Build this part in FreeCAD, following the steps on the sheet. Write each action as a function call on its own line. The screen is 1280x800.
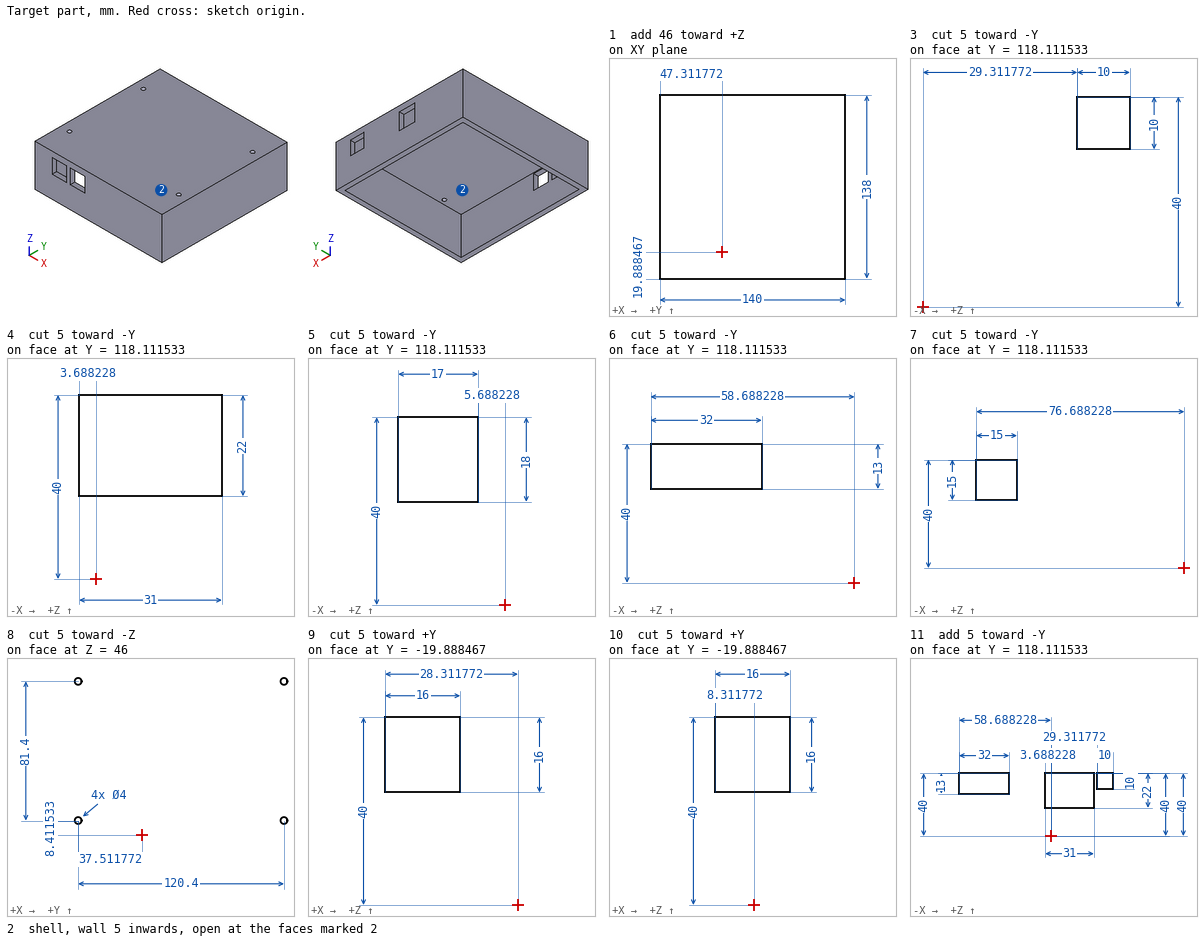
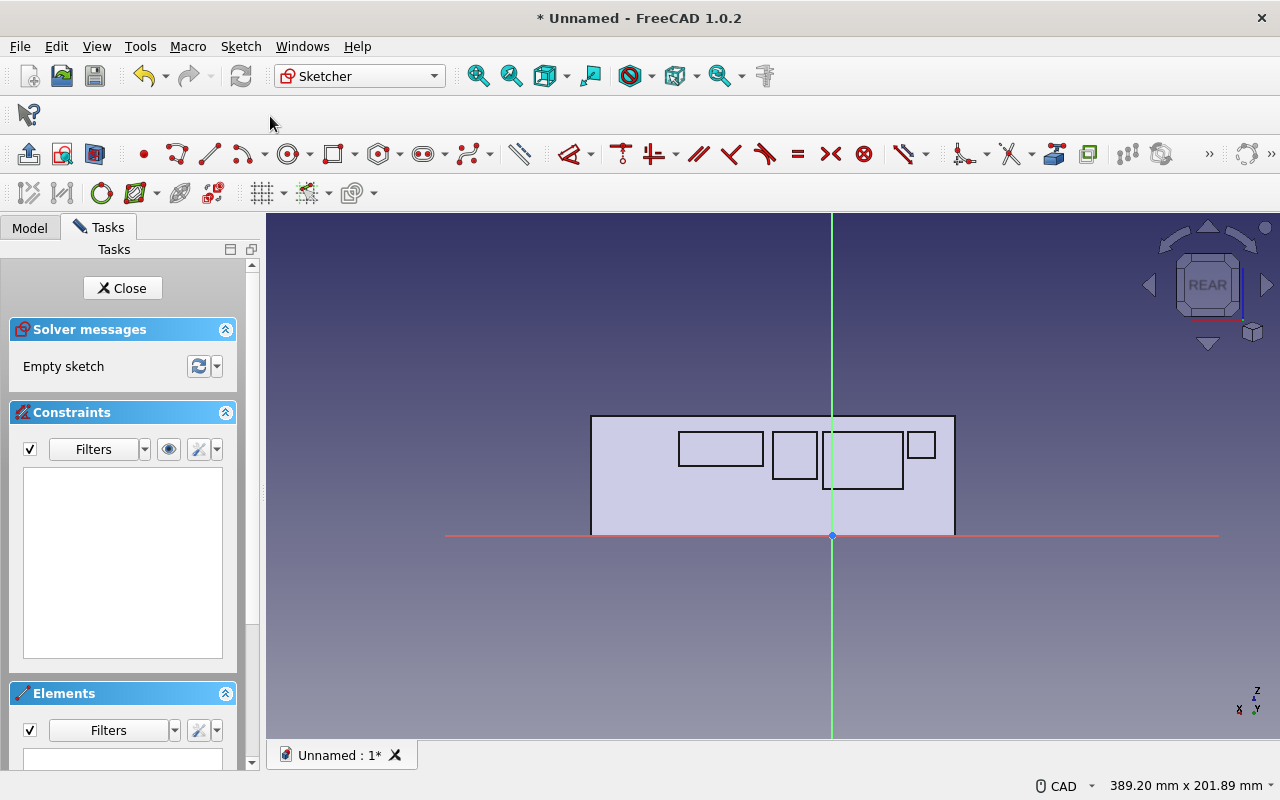
scroll(645, 448, up, 11)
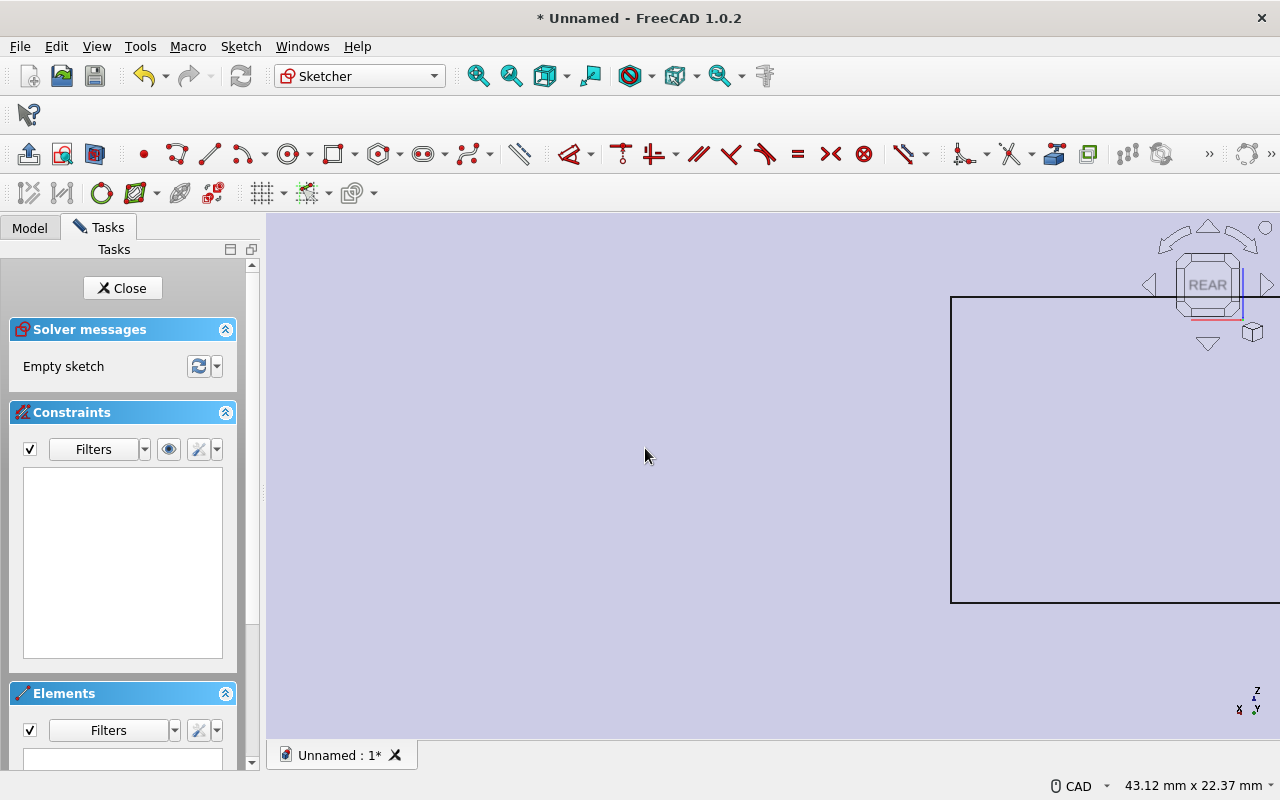
click(332, 154)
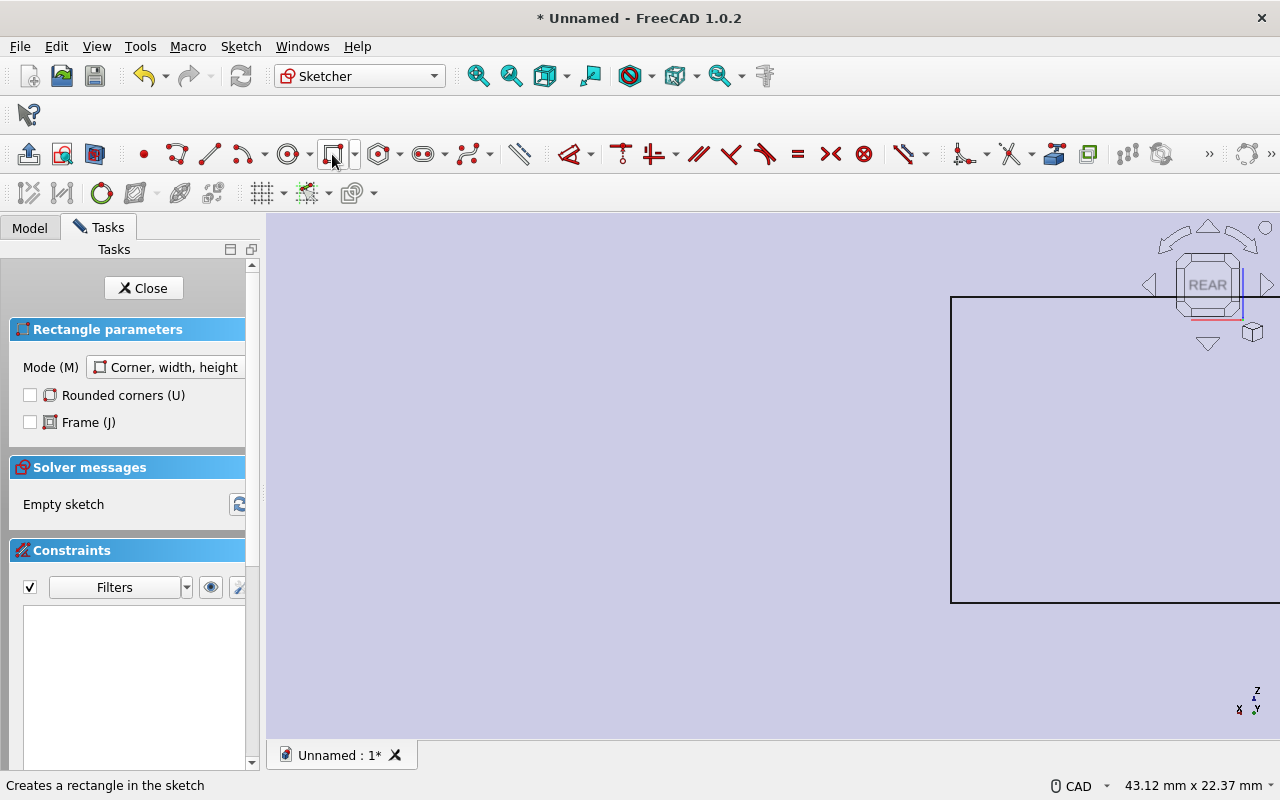
click(527, 297)
move(880, 650)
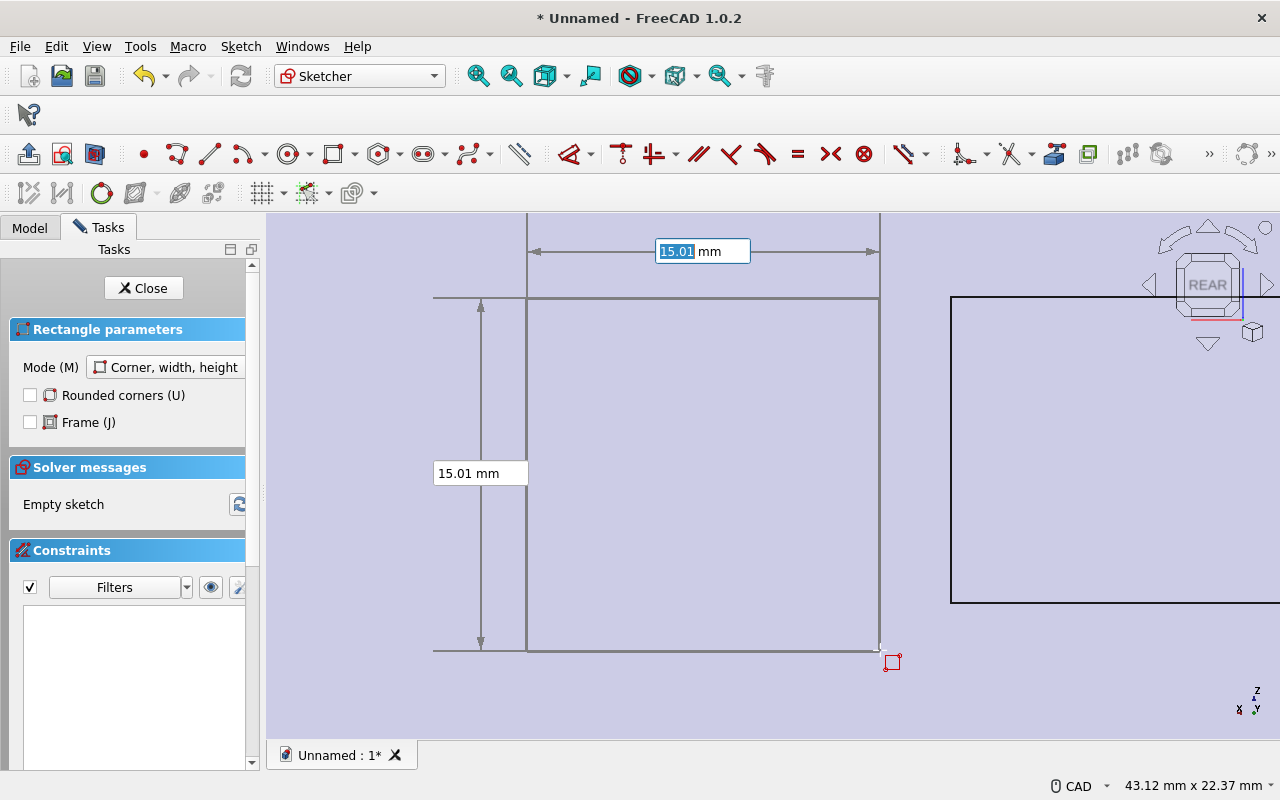
text(15)
key(Tab)
text(15)
key(Return)
key(Escape)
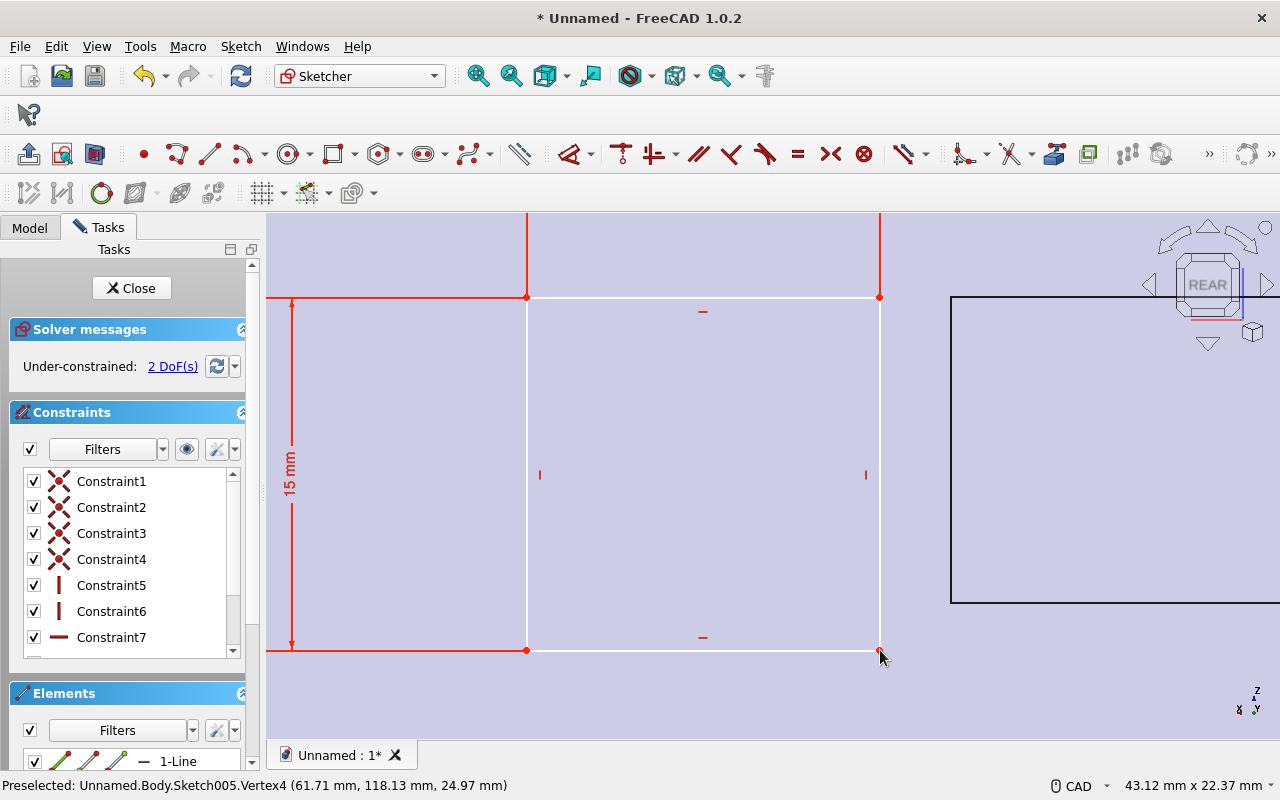
click(568, 154)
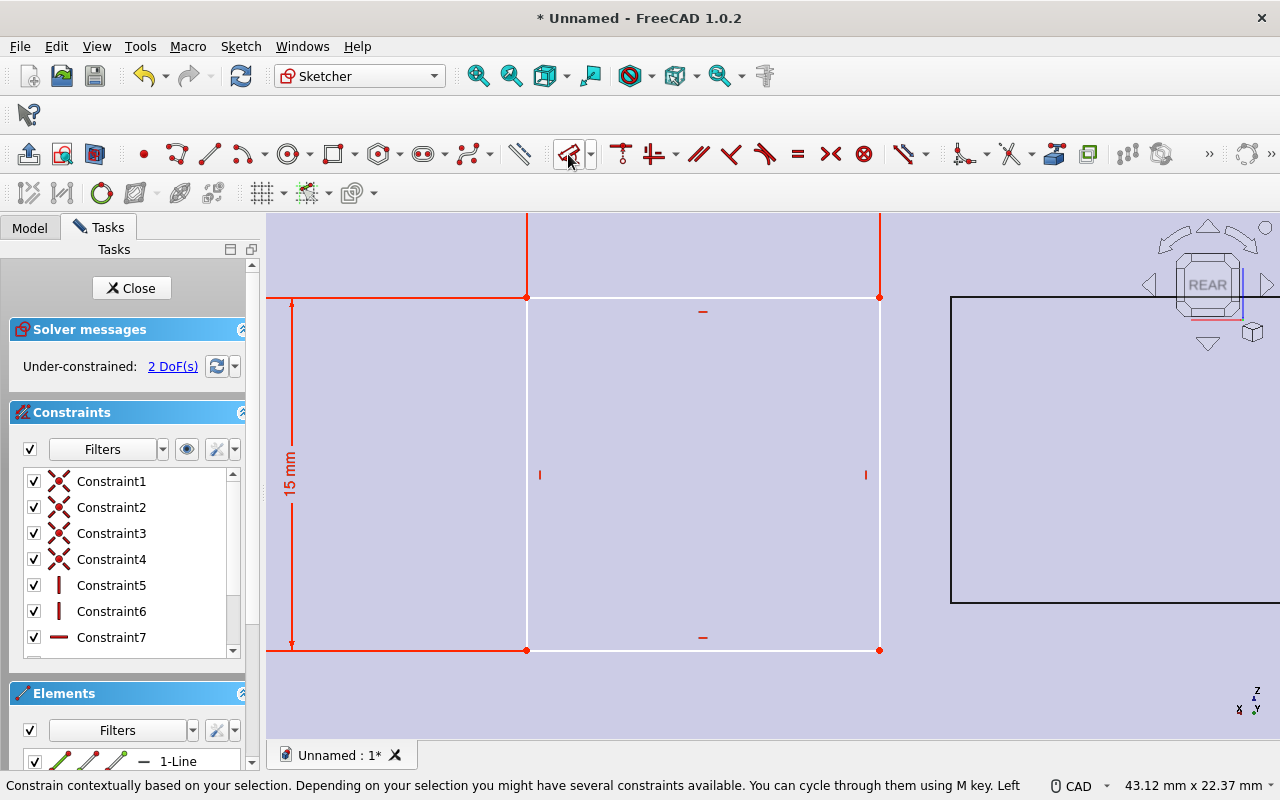
click(527, 298)
click(493, 505)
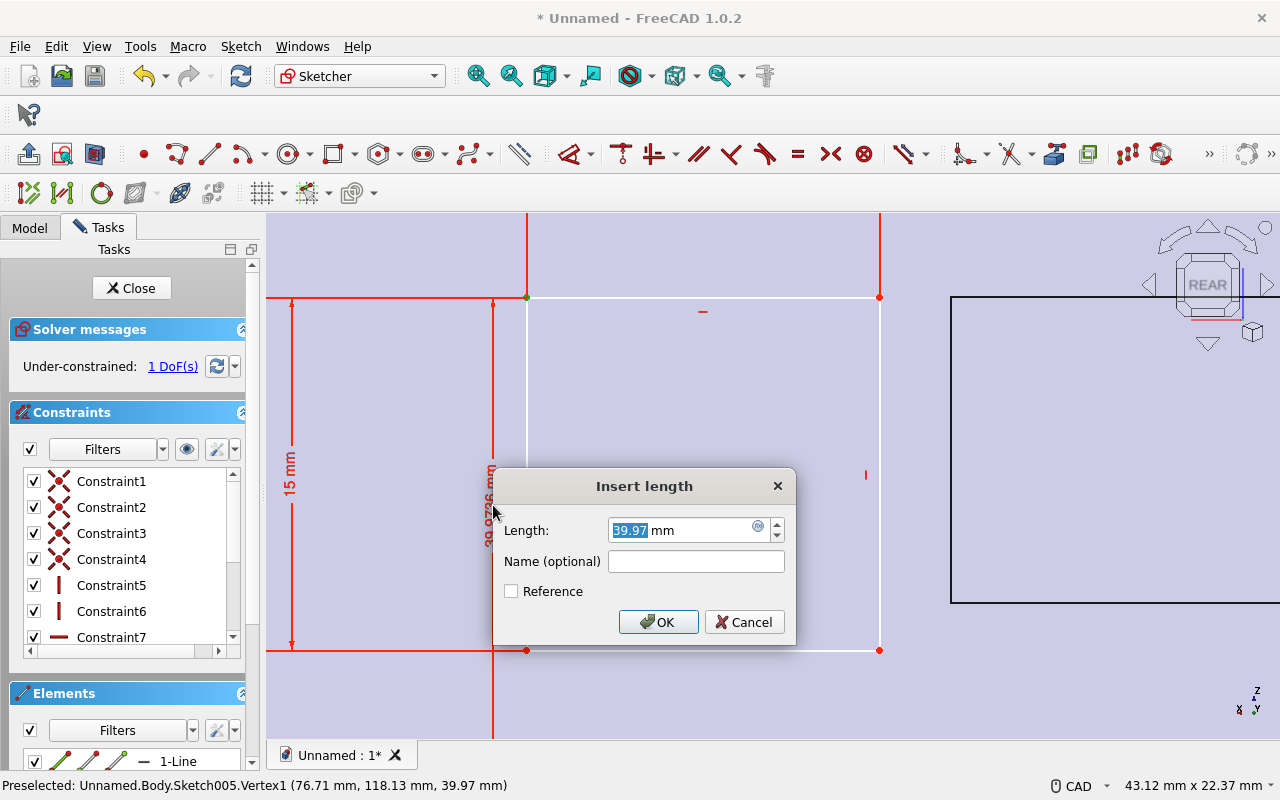
text(40)
key(Return)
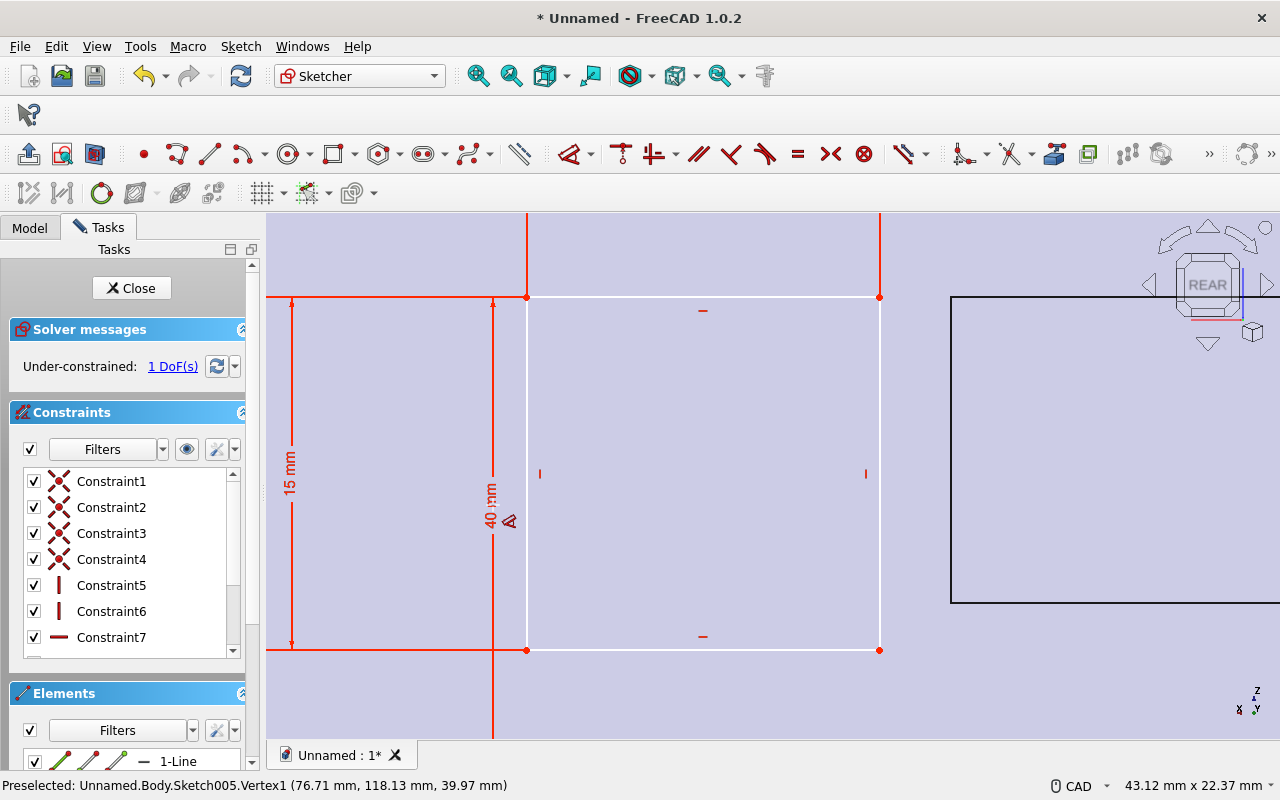
click(527, 297)
click(821, 263)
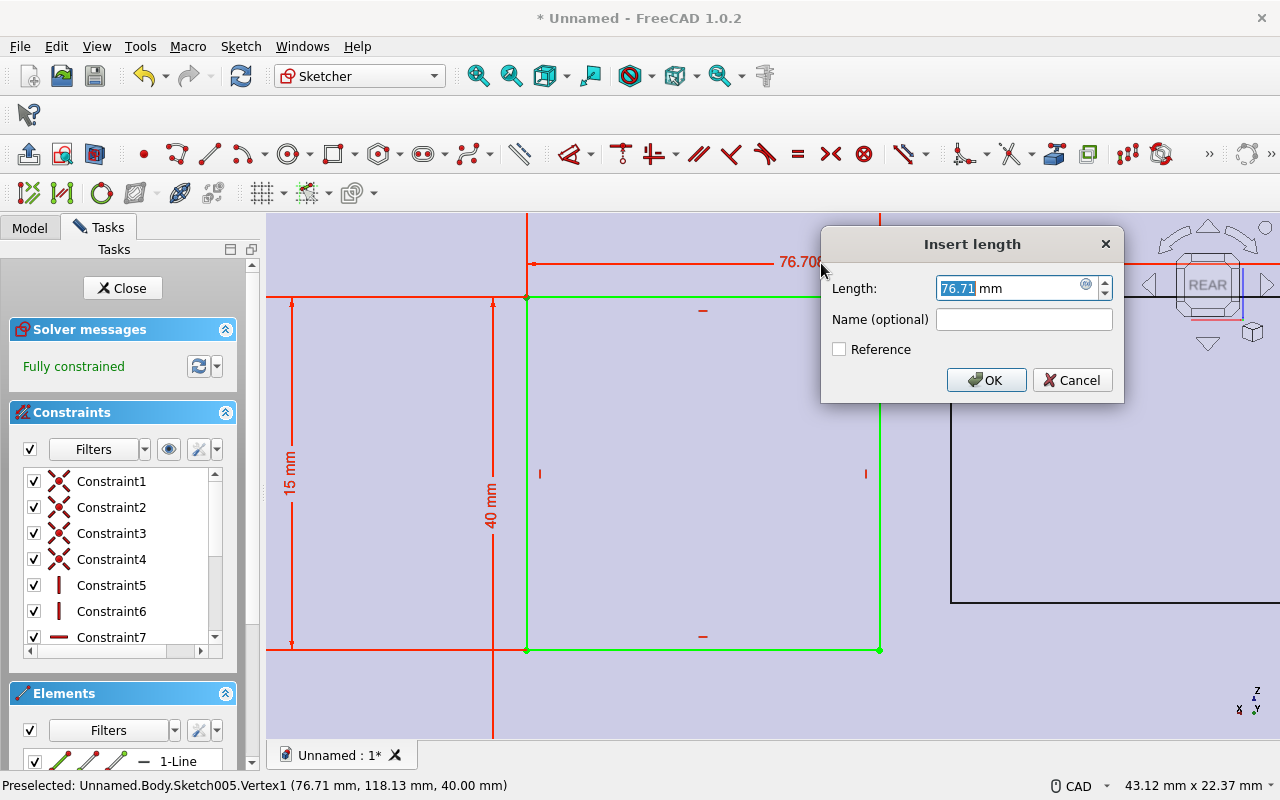
text(76.688228)
key(Return)
key(Escape)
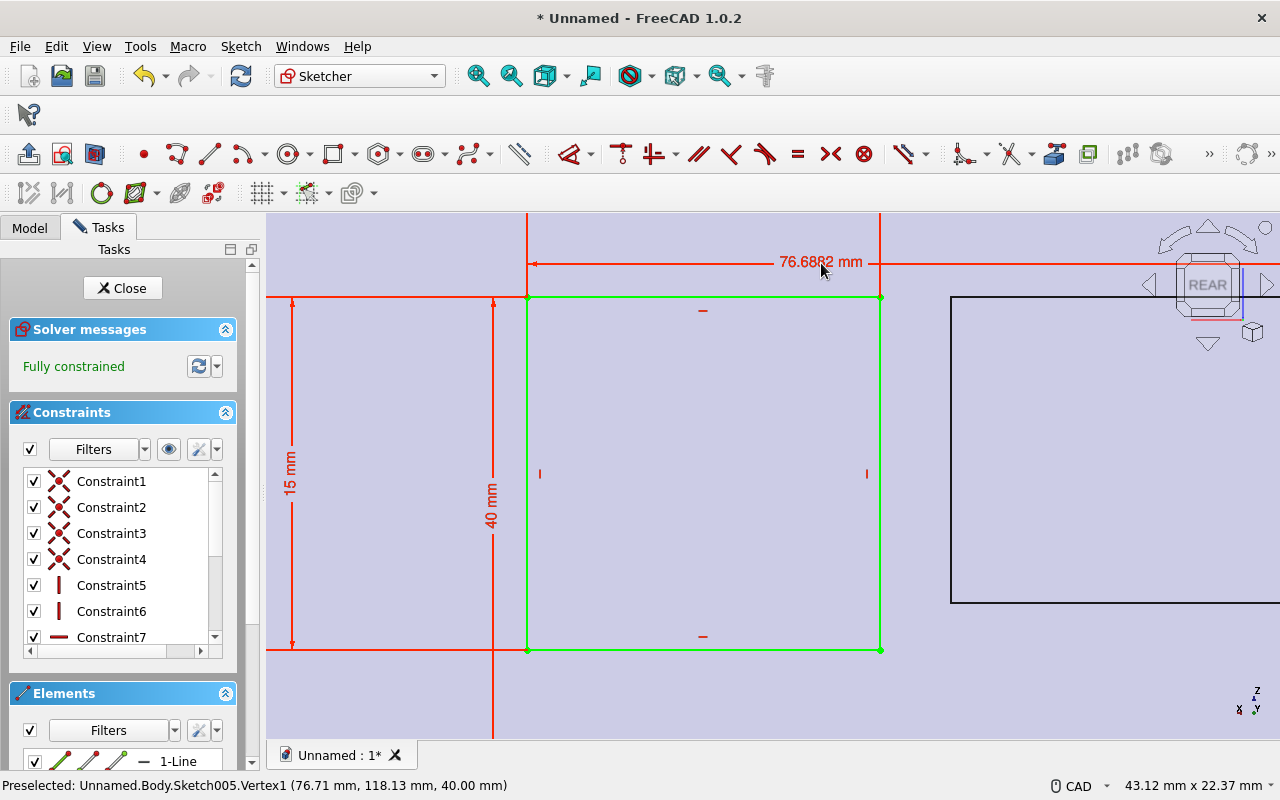
click(123, 288)